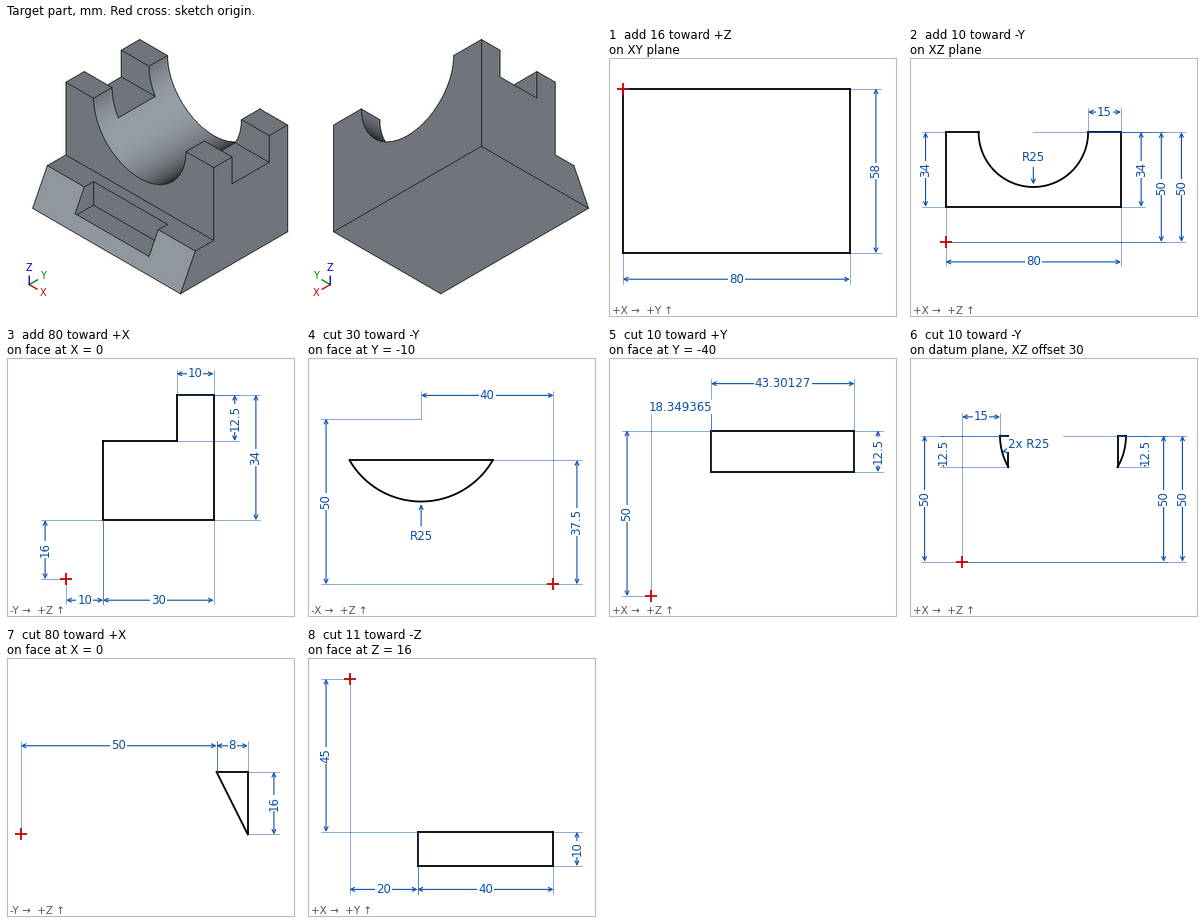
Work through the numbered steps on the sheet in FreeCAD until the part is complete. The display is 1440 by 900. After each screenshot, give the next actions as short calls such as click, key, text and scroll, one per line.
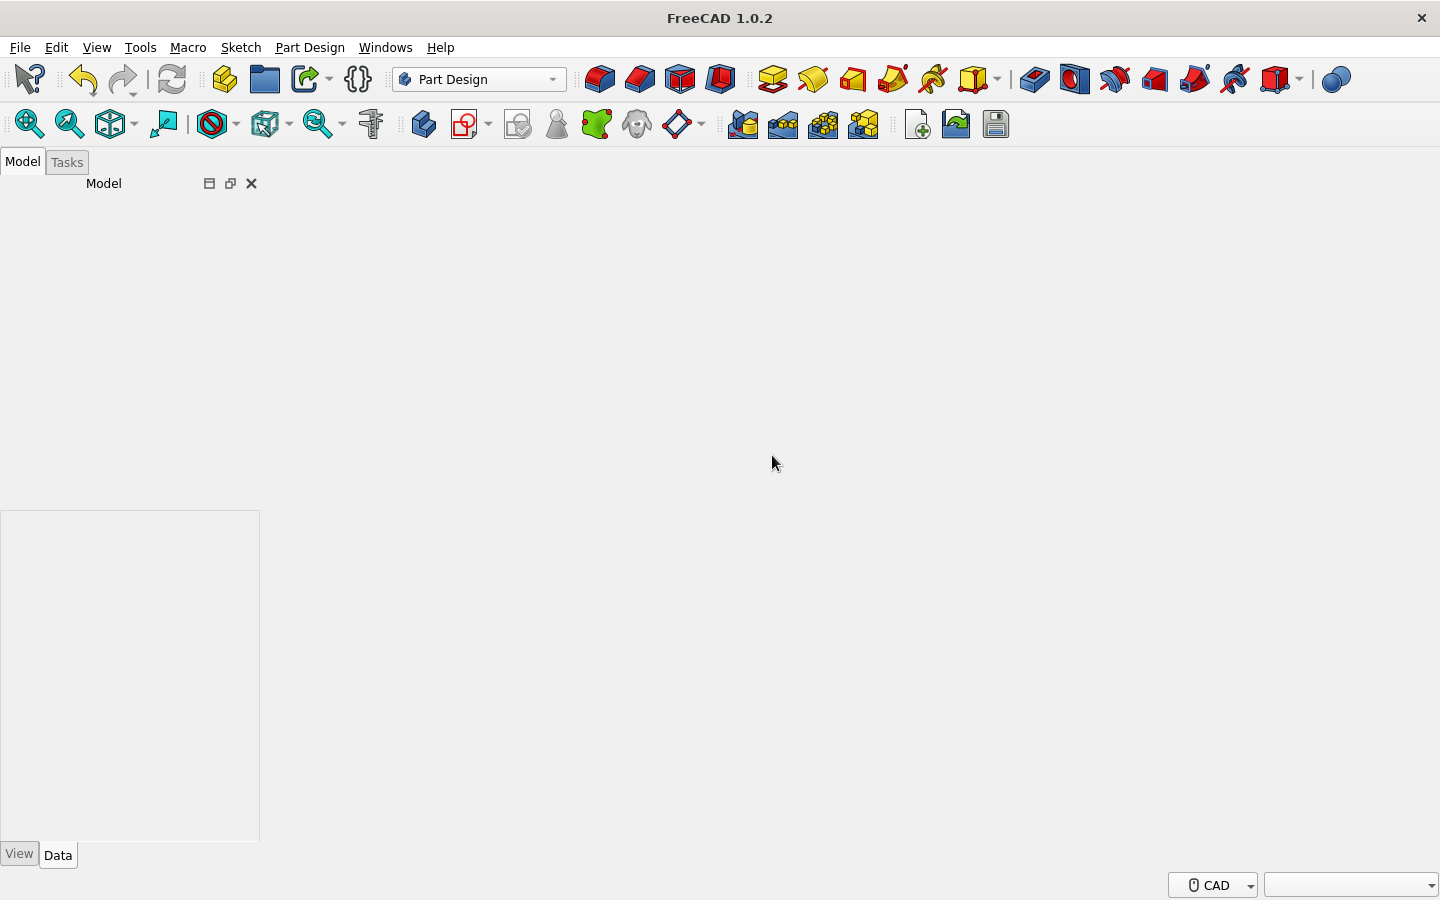
click(916, 124)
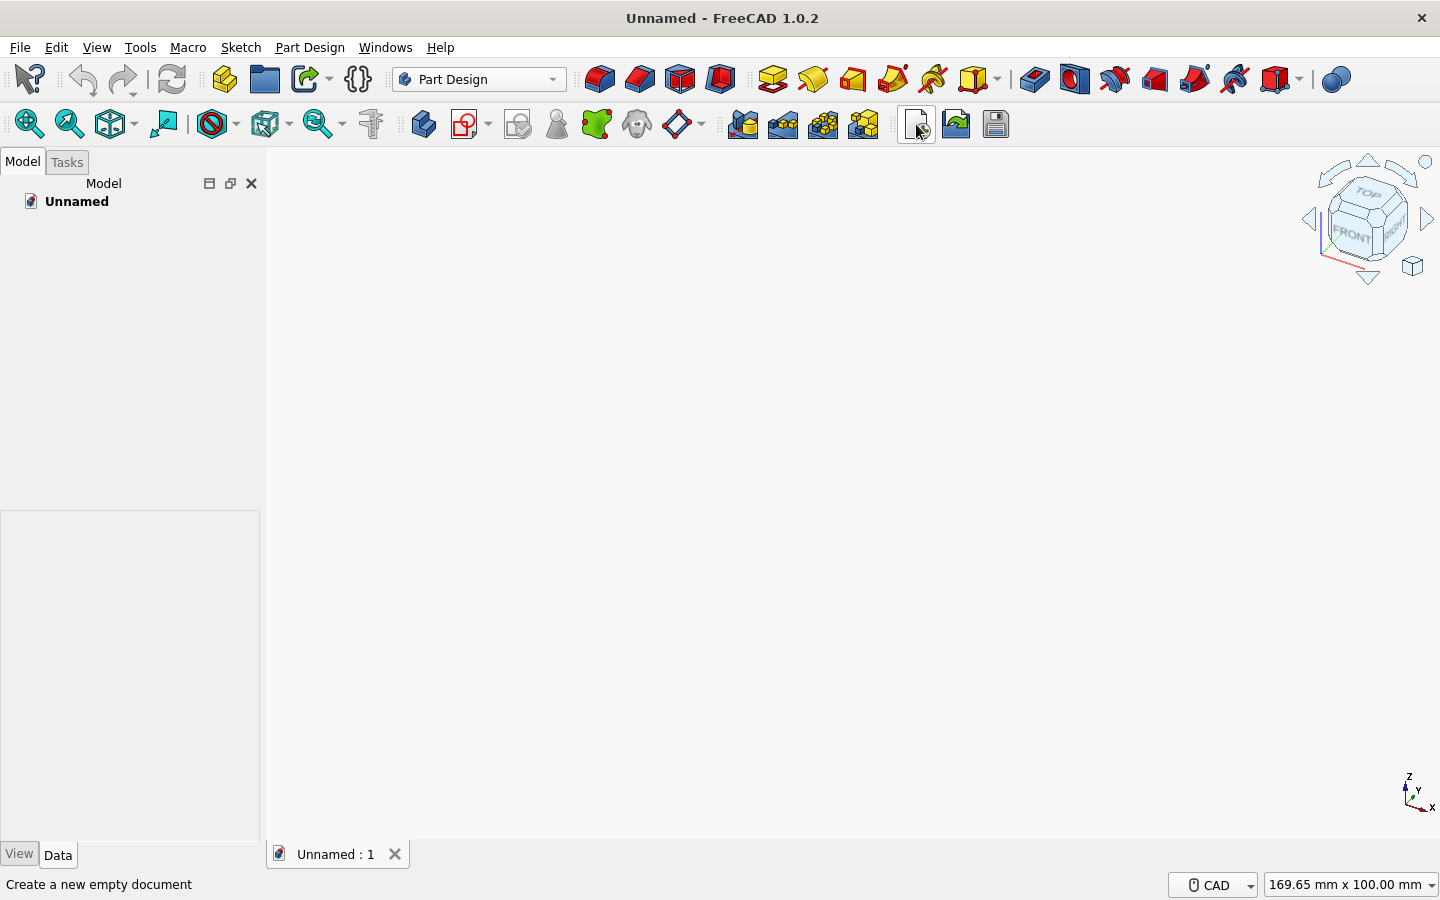
click(464, 124)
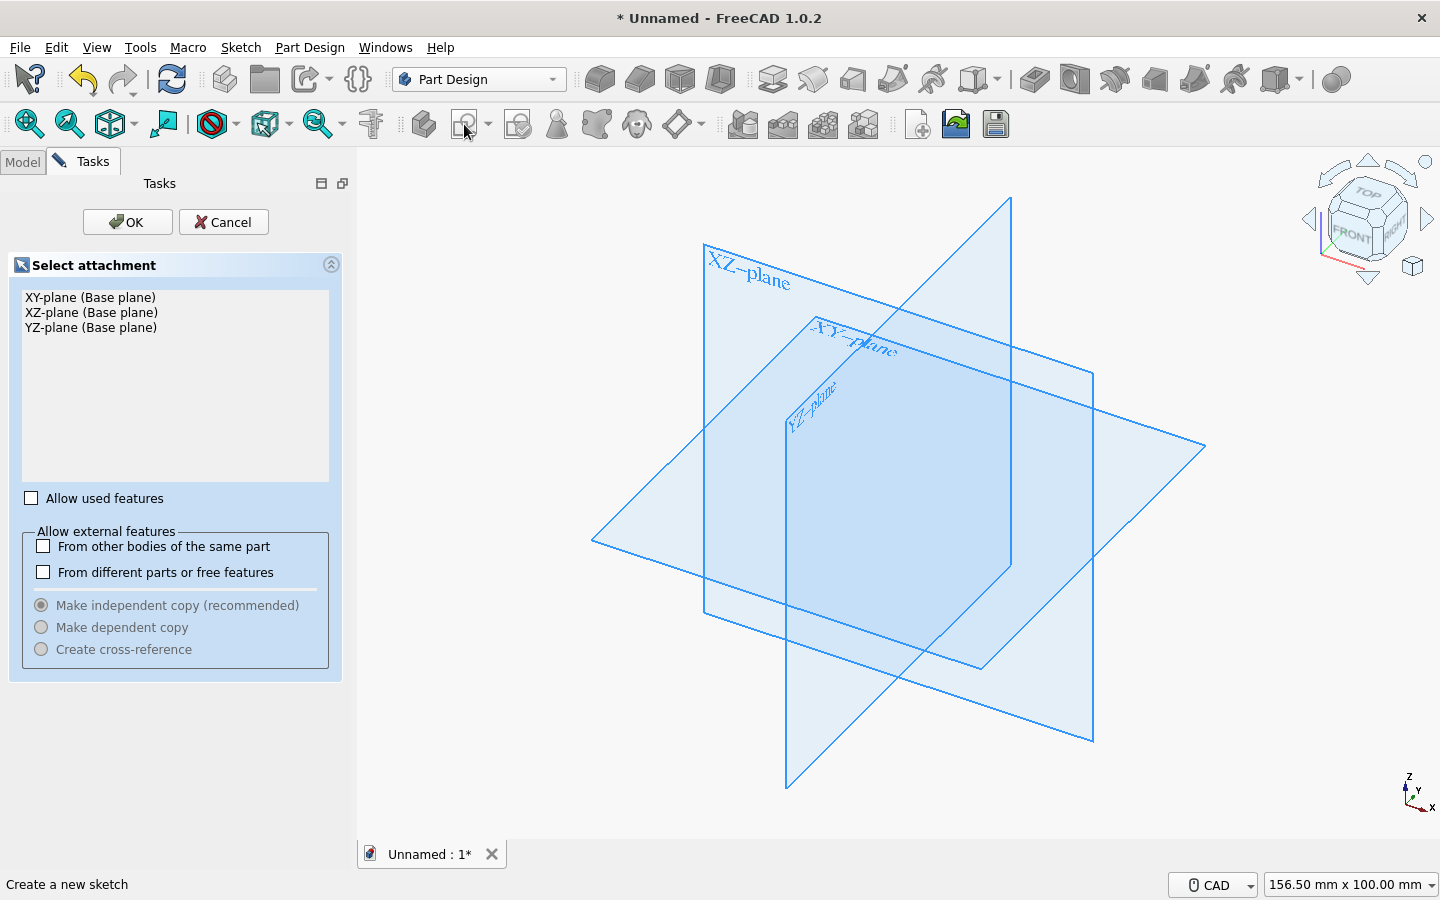
click(82, 298)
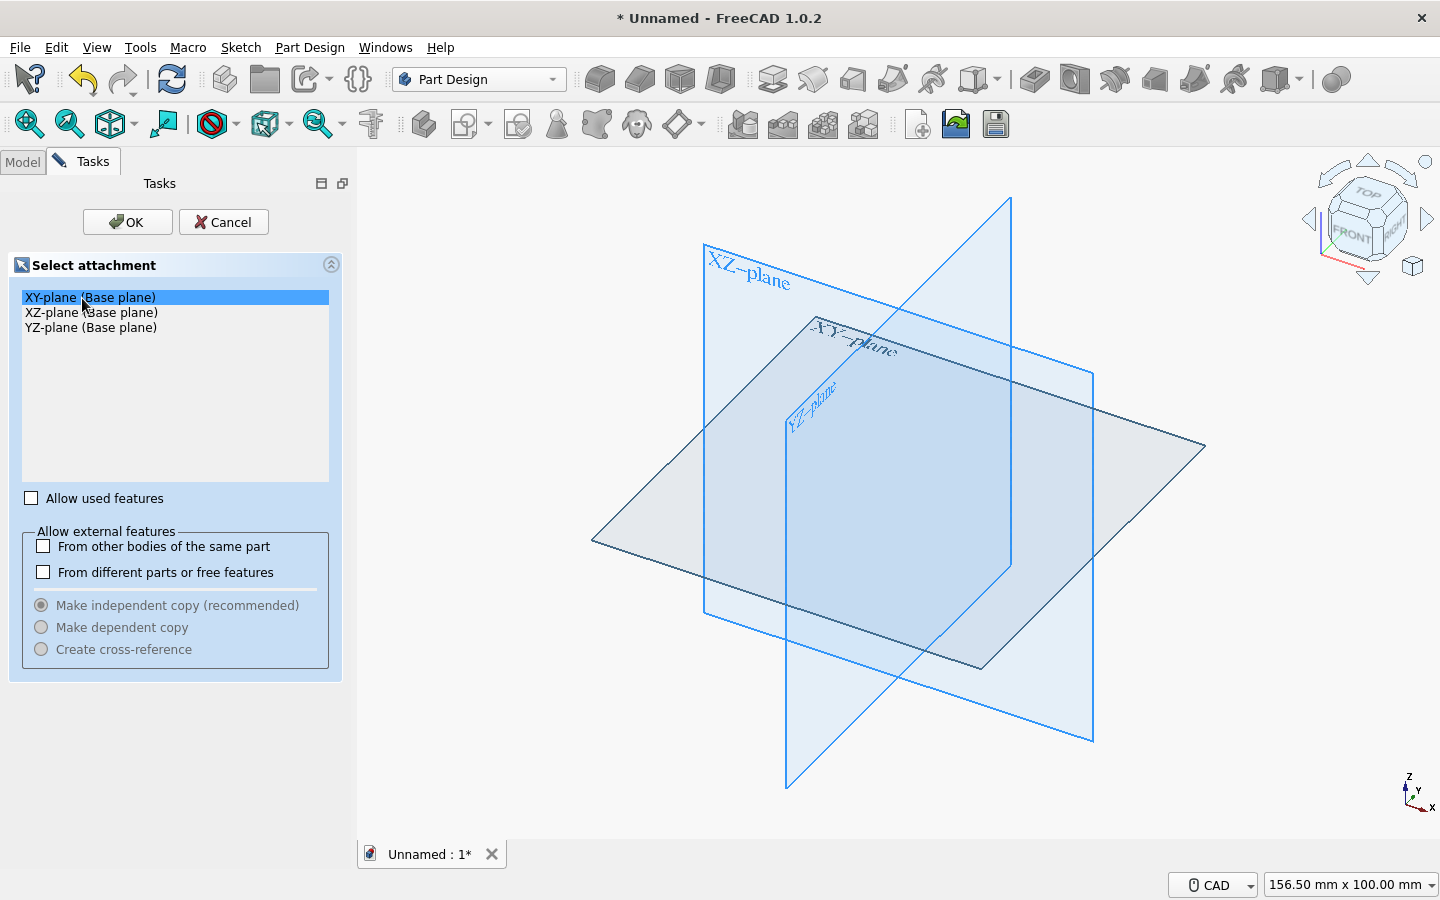
click(128, 222)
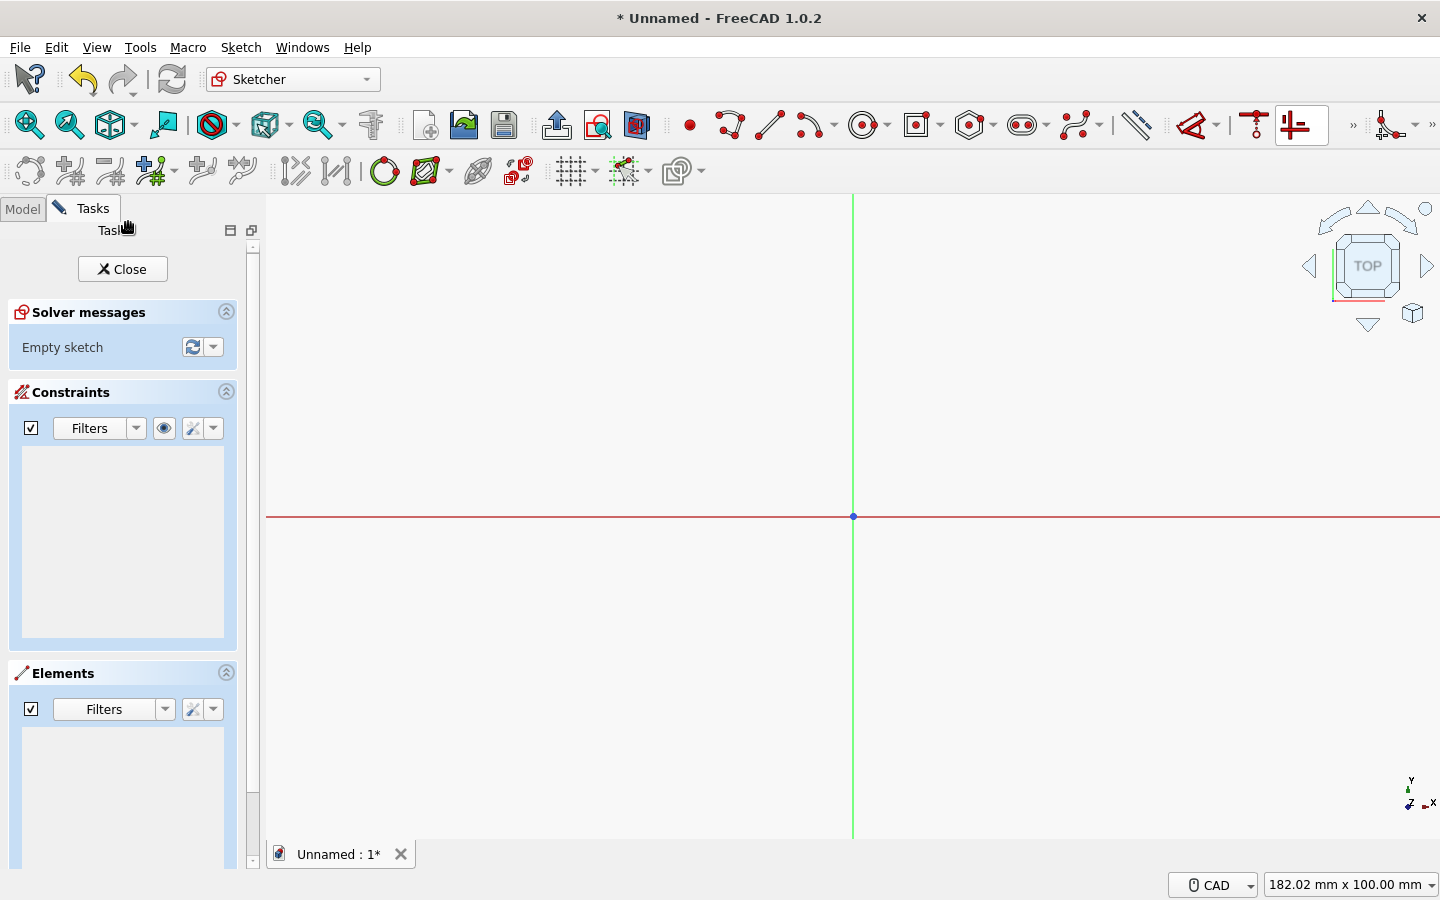
scroll(294, 222, down, 1)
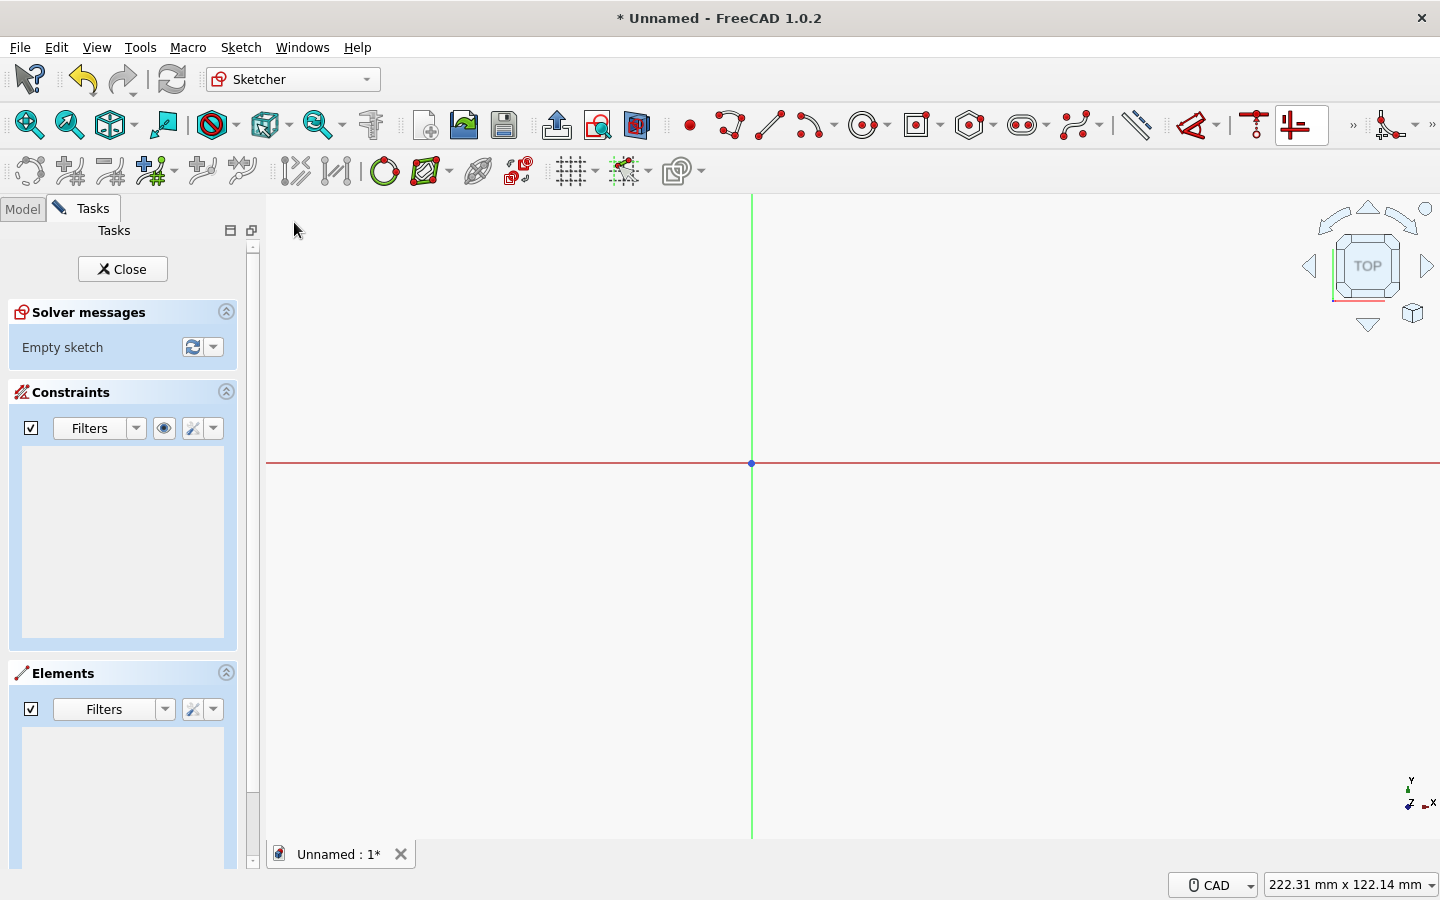
scroll(1275, 811, up, 2)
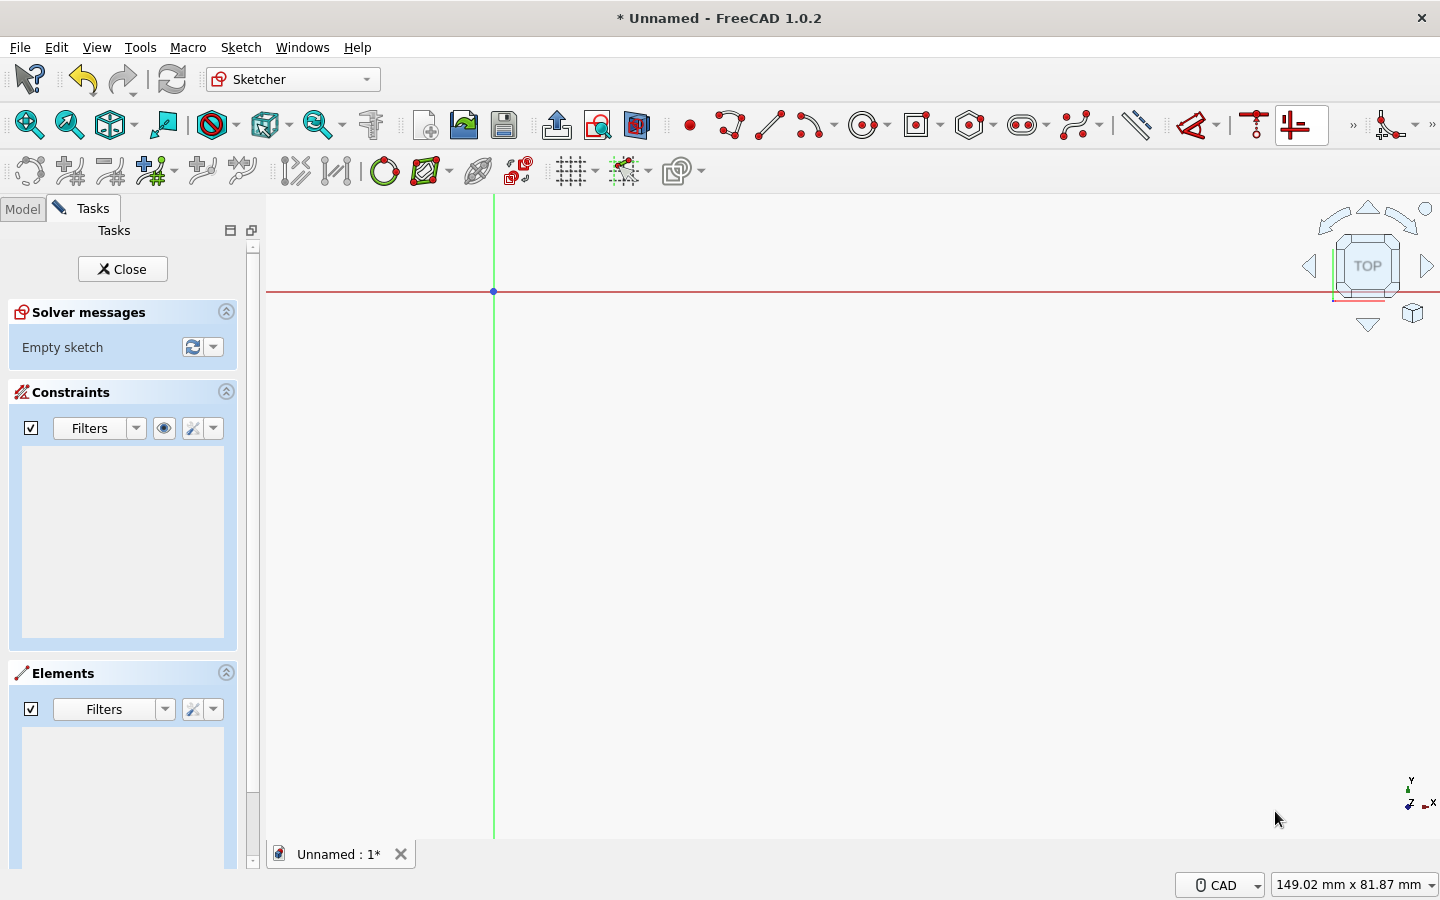
click(942, 126)